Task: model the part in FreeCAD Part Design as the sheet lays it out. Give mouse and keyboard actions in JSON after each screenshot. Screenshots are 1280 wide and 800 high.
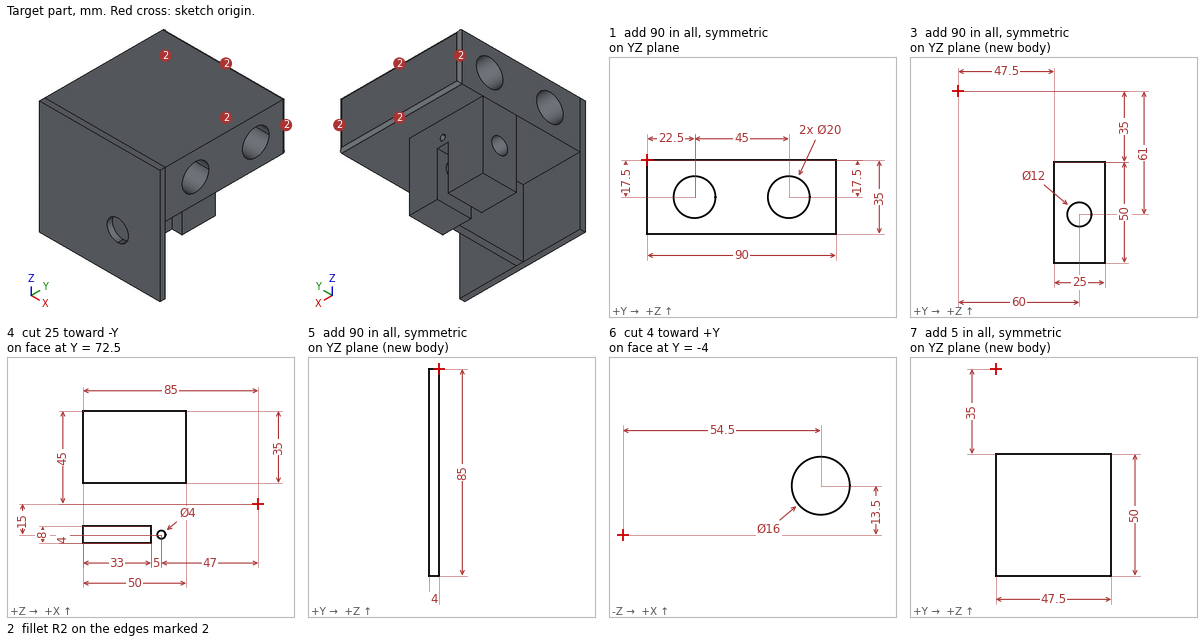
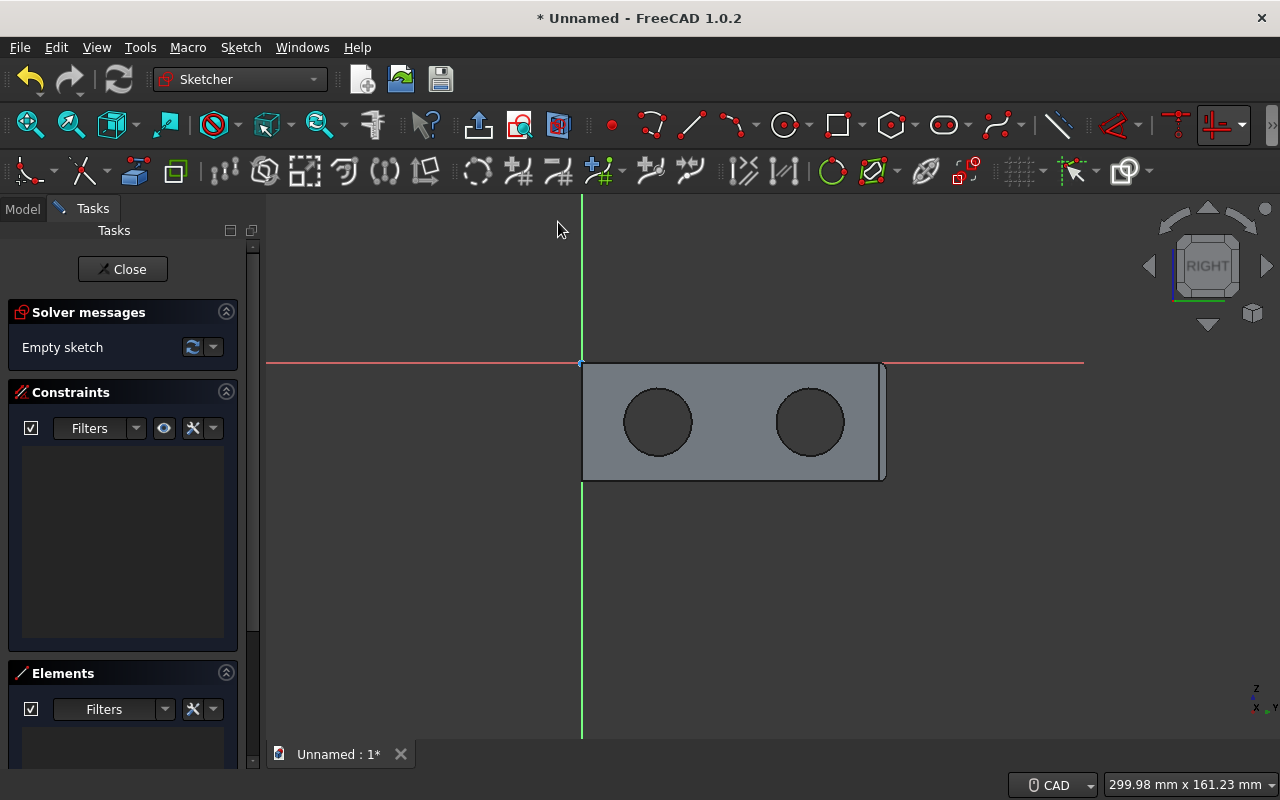
{"action": "left_click", "coordinate": [838, 126]}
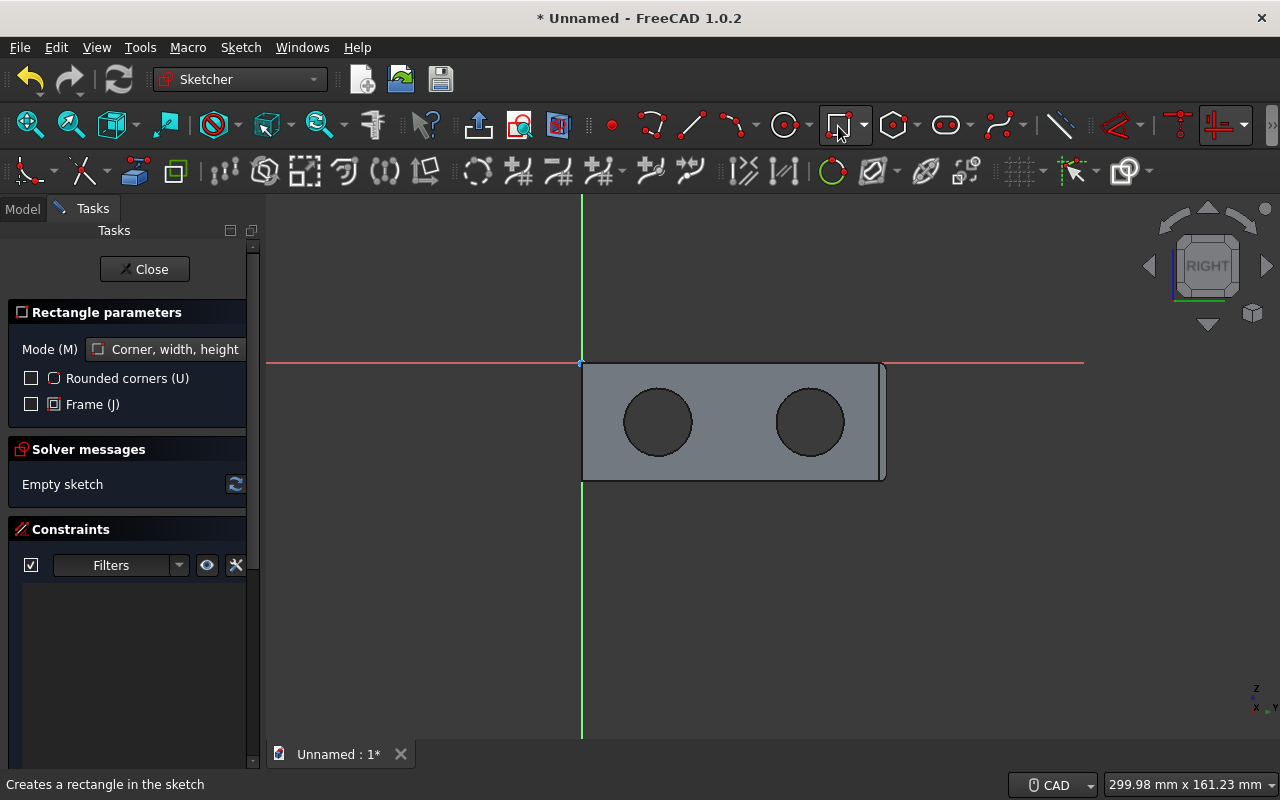
{"action": "left_click", "coordinate": [743, 481]}
{"action": "mouse_move", "coordinate": [827, 650]}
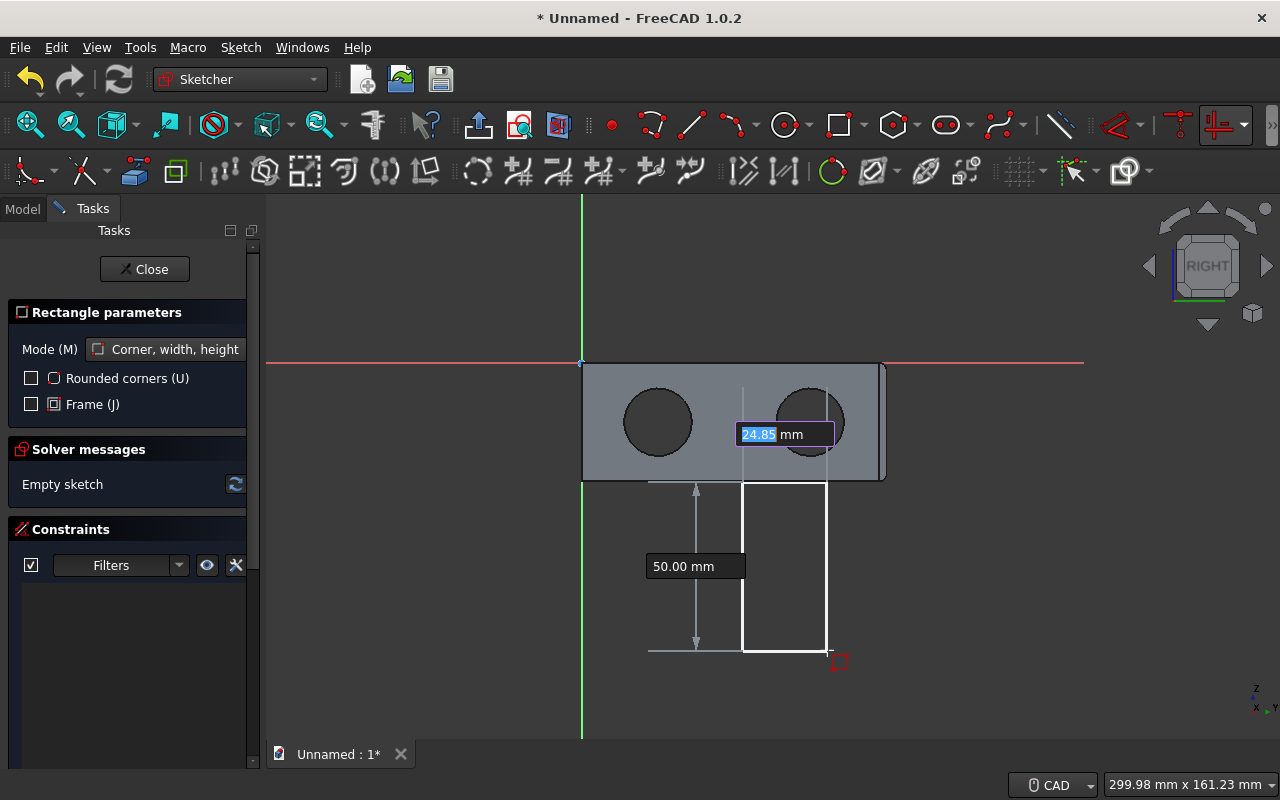
{"action": "type", "text": "25"}
{"action": "key", "text": "Tab"}
{"action": "type", "text": "50"}
{"action": "key", "text": "Return"}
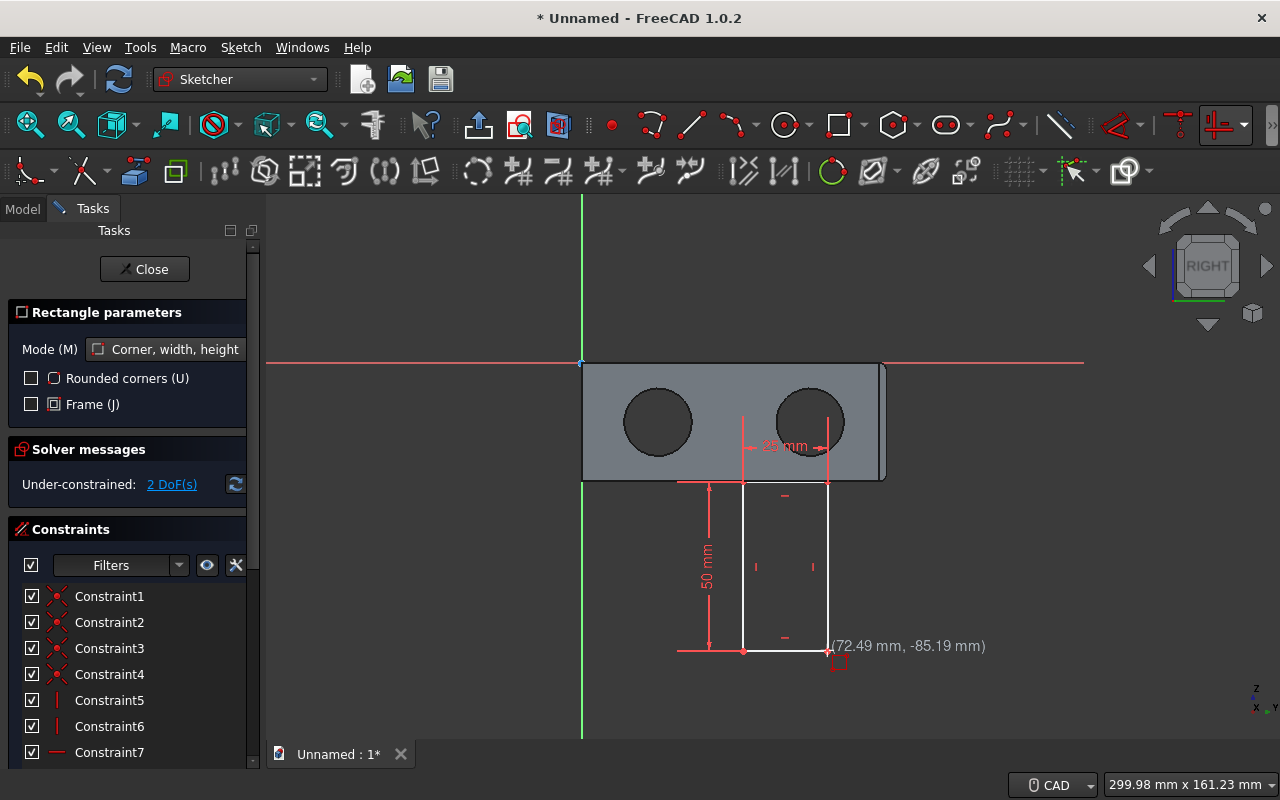
{"action": "left_click", "coordinate": [786, 126]}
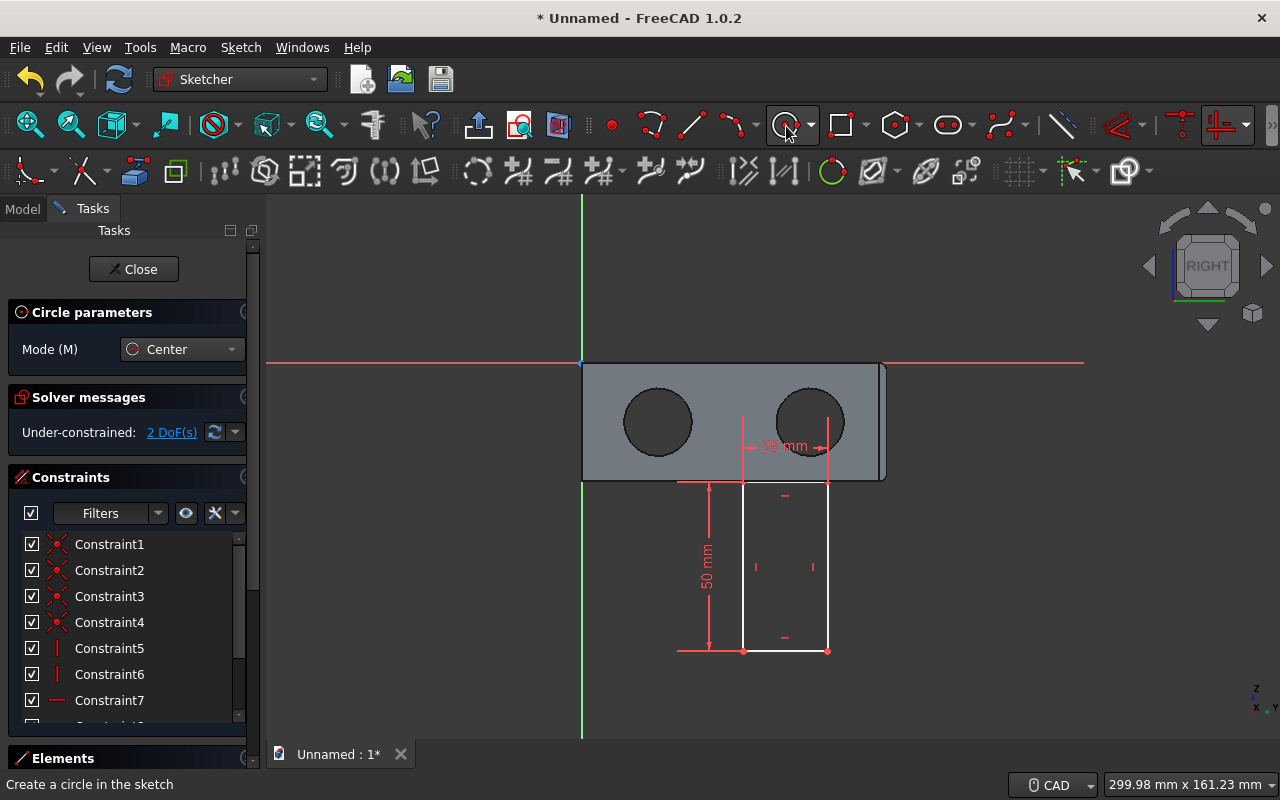
{"action": "left_click", "coordinate": [785, 569]}
{"action": "mouse_move", "coordinate": [799, 555]}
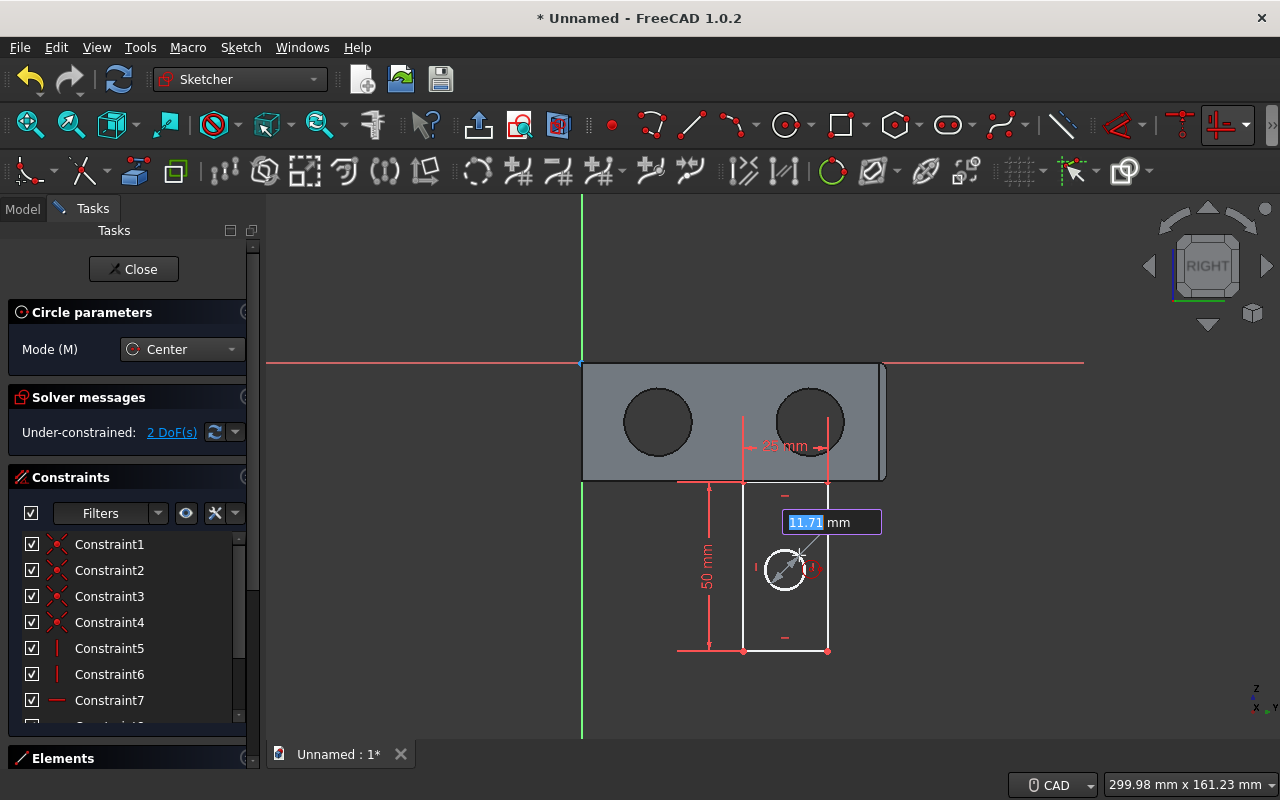
{"action": "type", "text": "12"}
{"action": "key", "text": "Return"}
{"action": "key", "text": "Escape"}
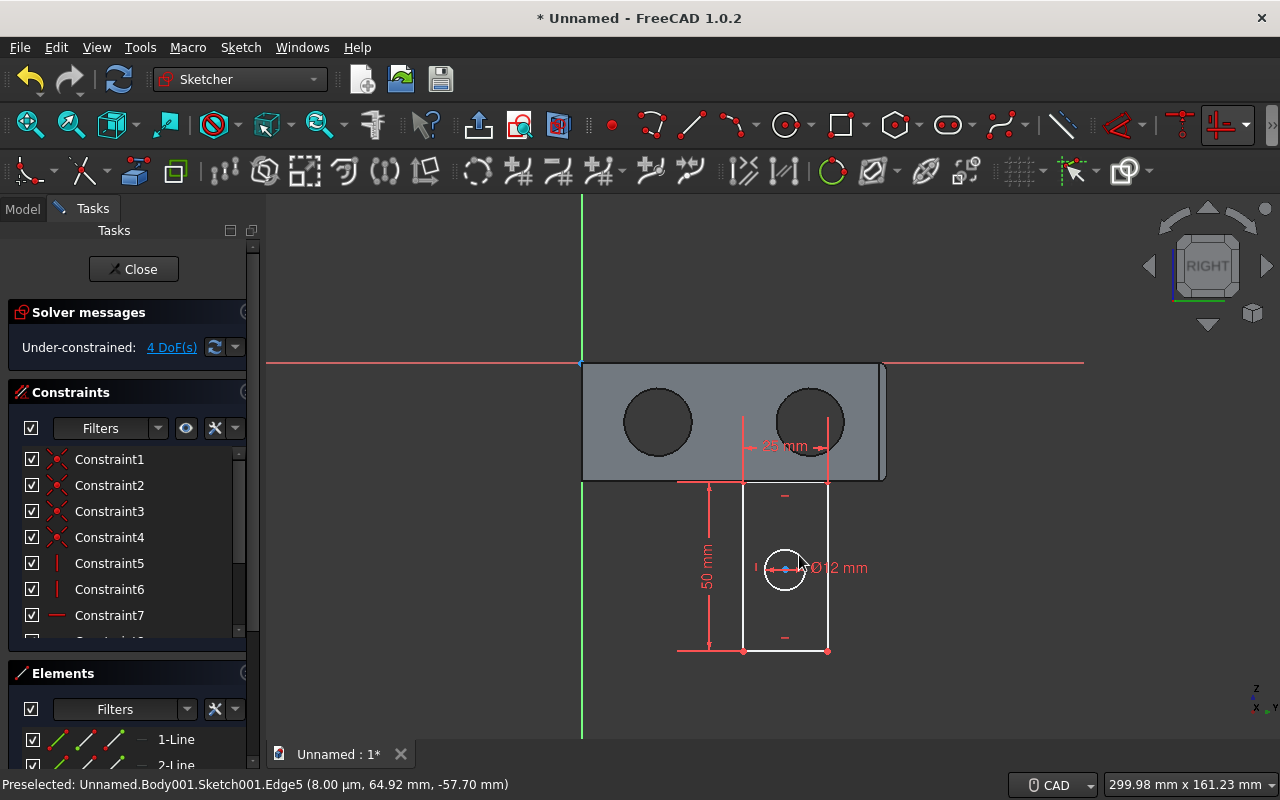
{"action": "left_click", "coordinate": [1118, 126]}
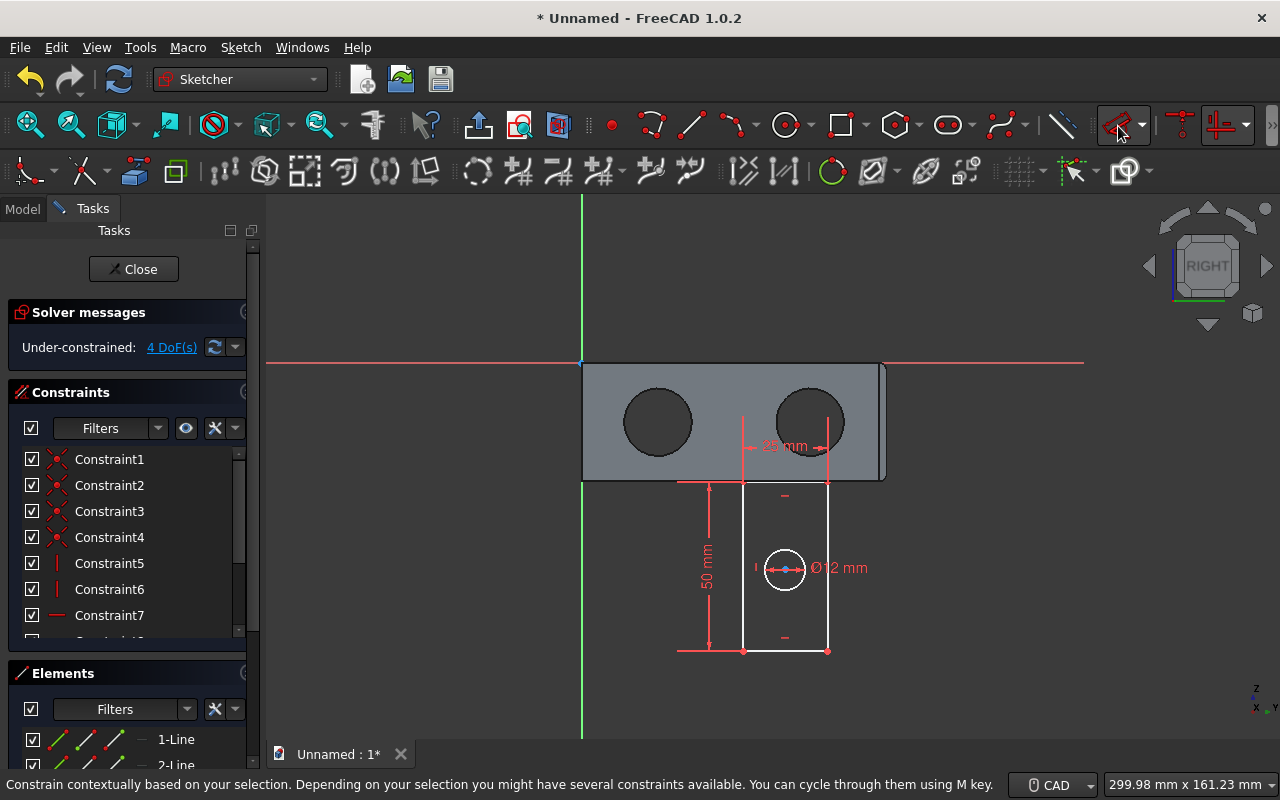
{"action": "left_click", "coordinate": [785, 570]}
{"action": "left_click", "coordinate": [683, 329]}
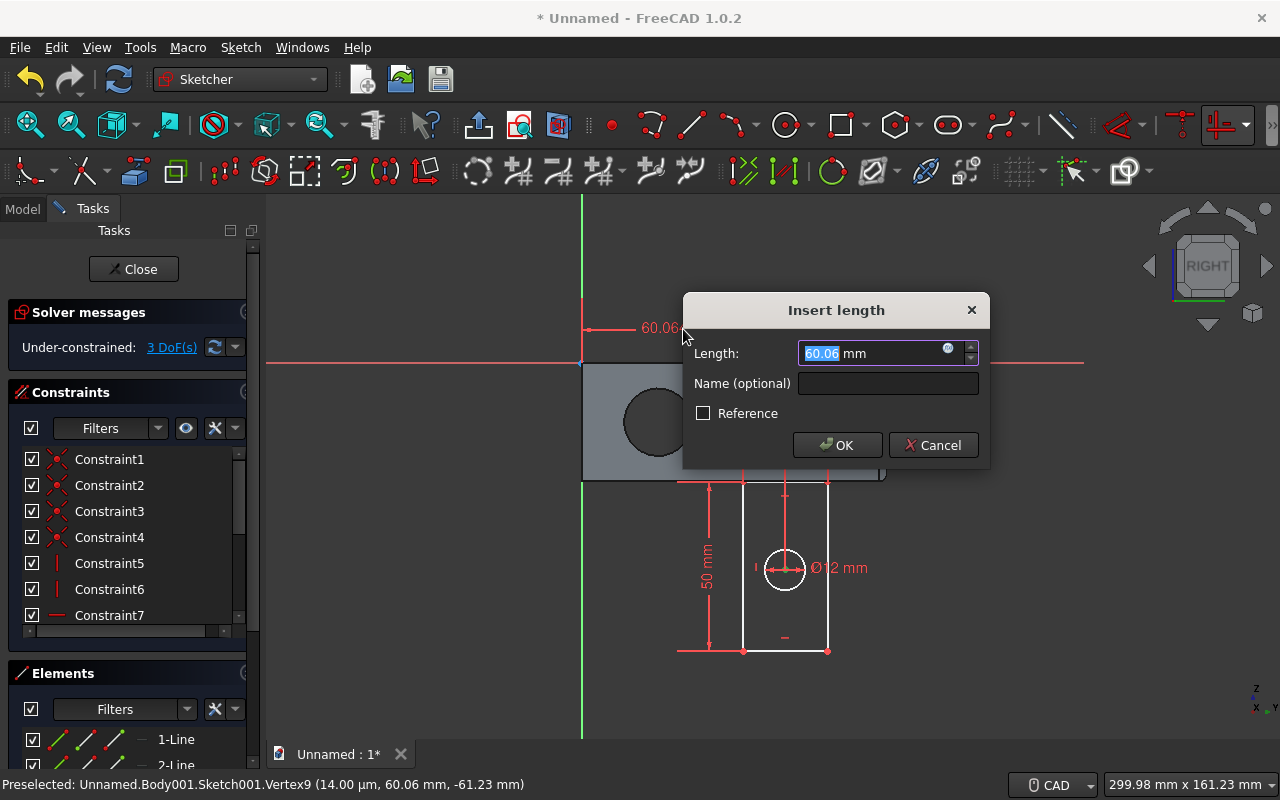
{"action": "type", "text": "60"}
{"action": "key", "text": "Return"}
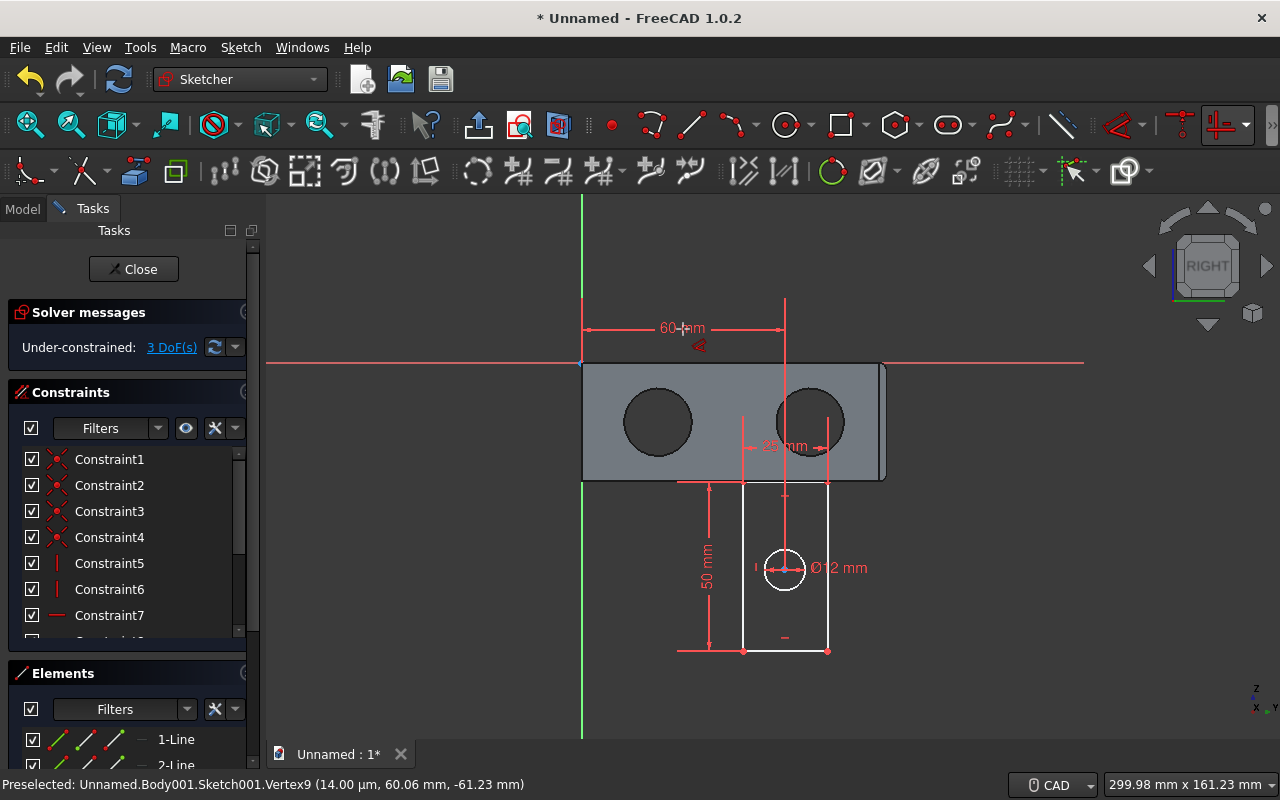
{"action": "left_click", "coordinate": [785, 570]}
{"action": "left_click", "coordinate": [548, 467]}